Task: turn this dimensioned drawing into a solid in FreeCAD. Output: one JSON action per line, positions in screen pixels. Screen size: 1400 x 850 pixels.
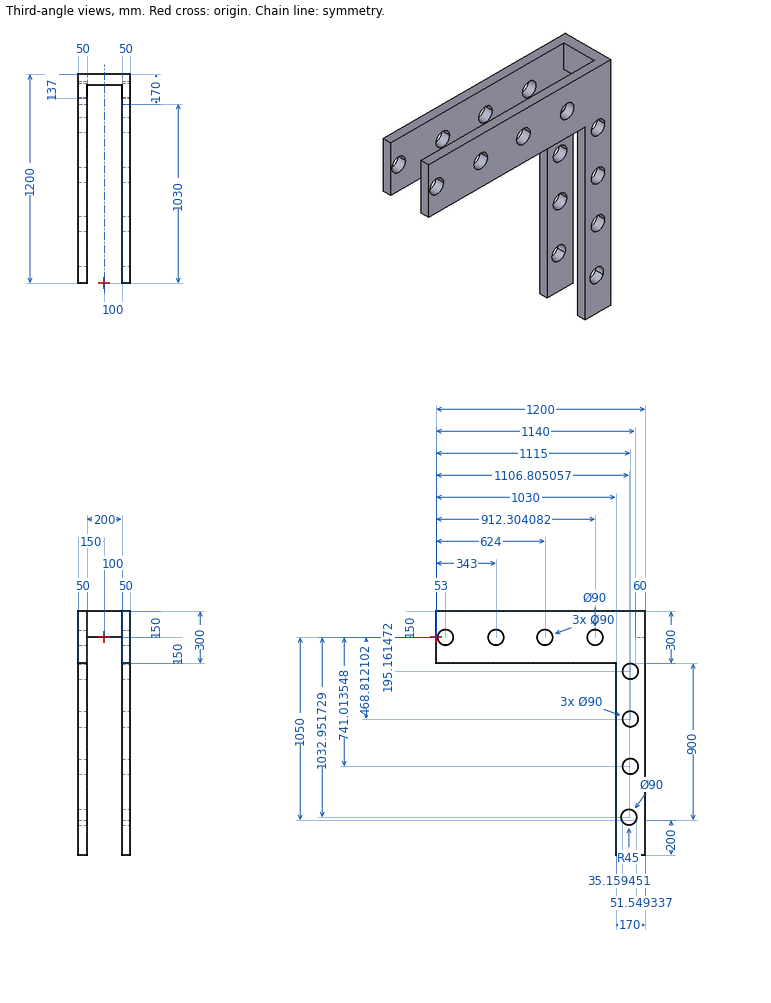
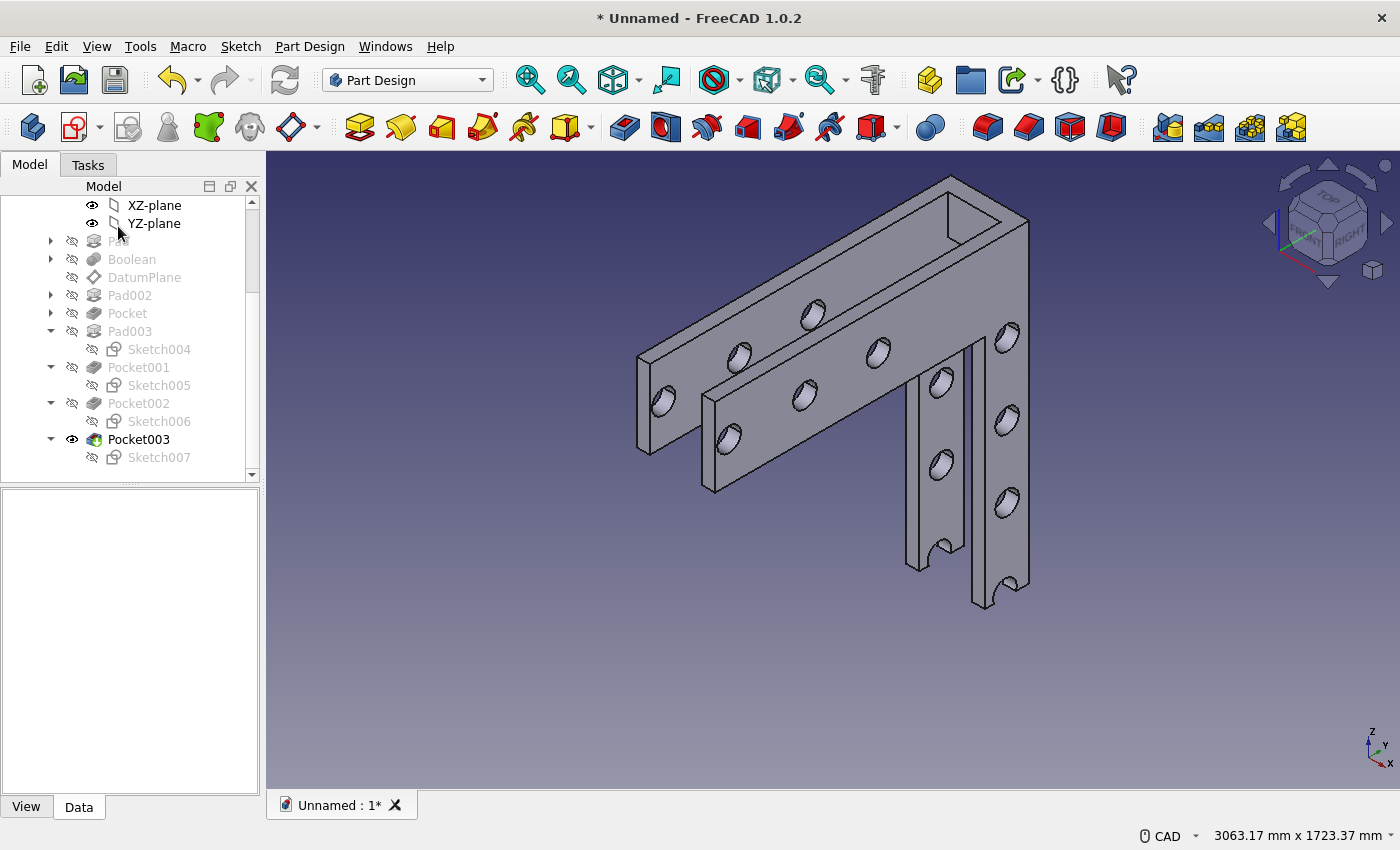
{"action": "key", "text": "6"}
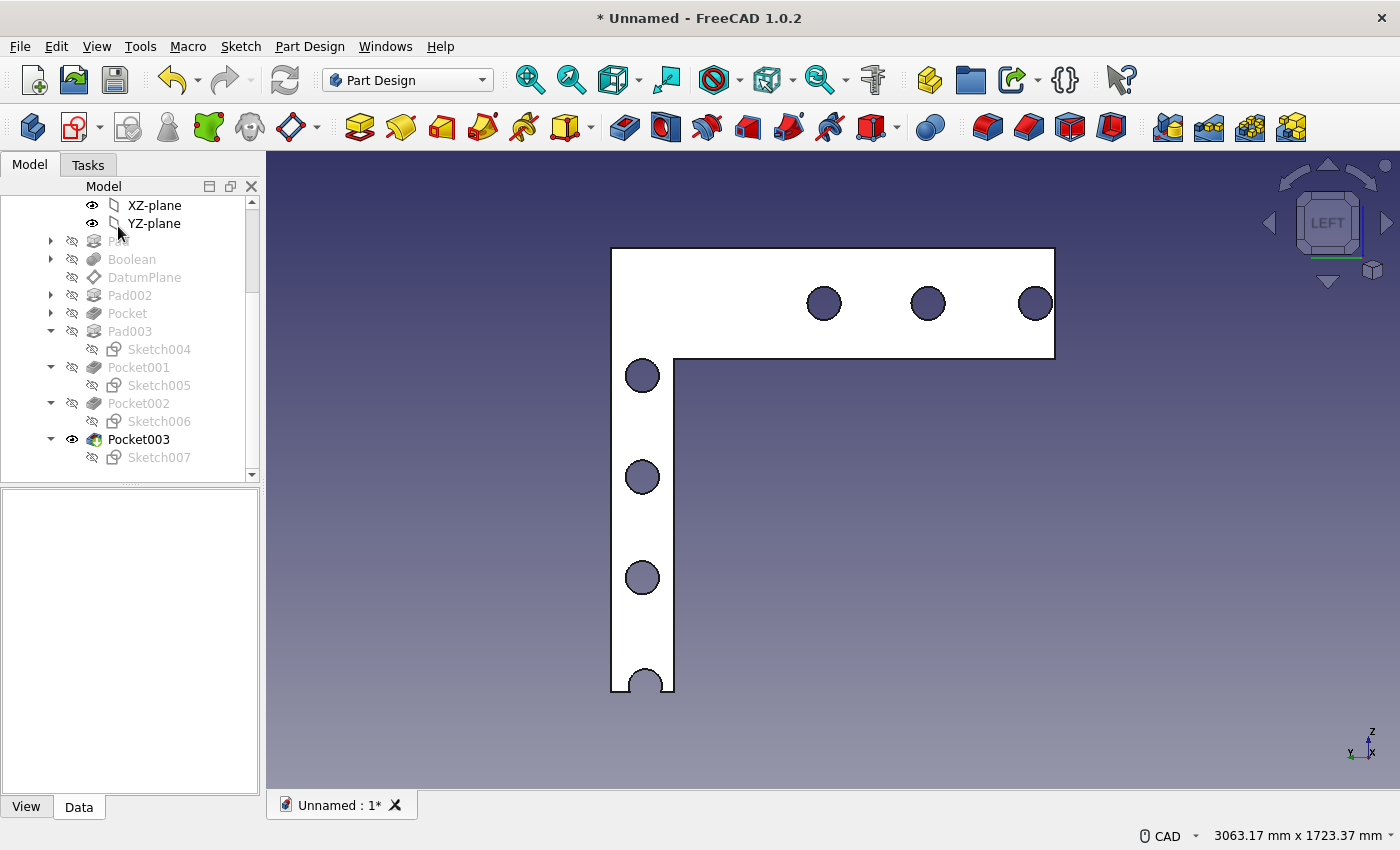
{"action": "left_click", "coordinate": [770, 279]}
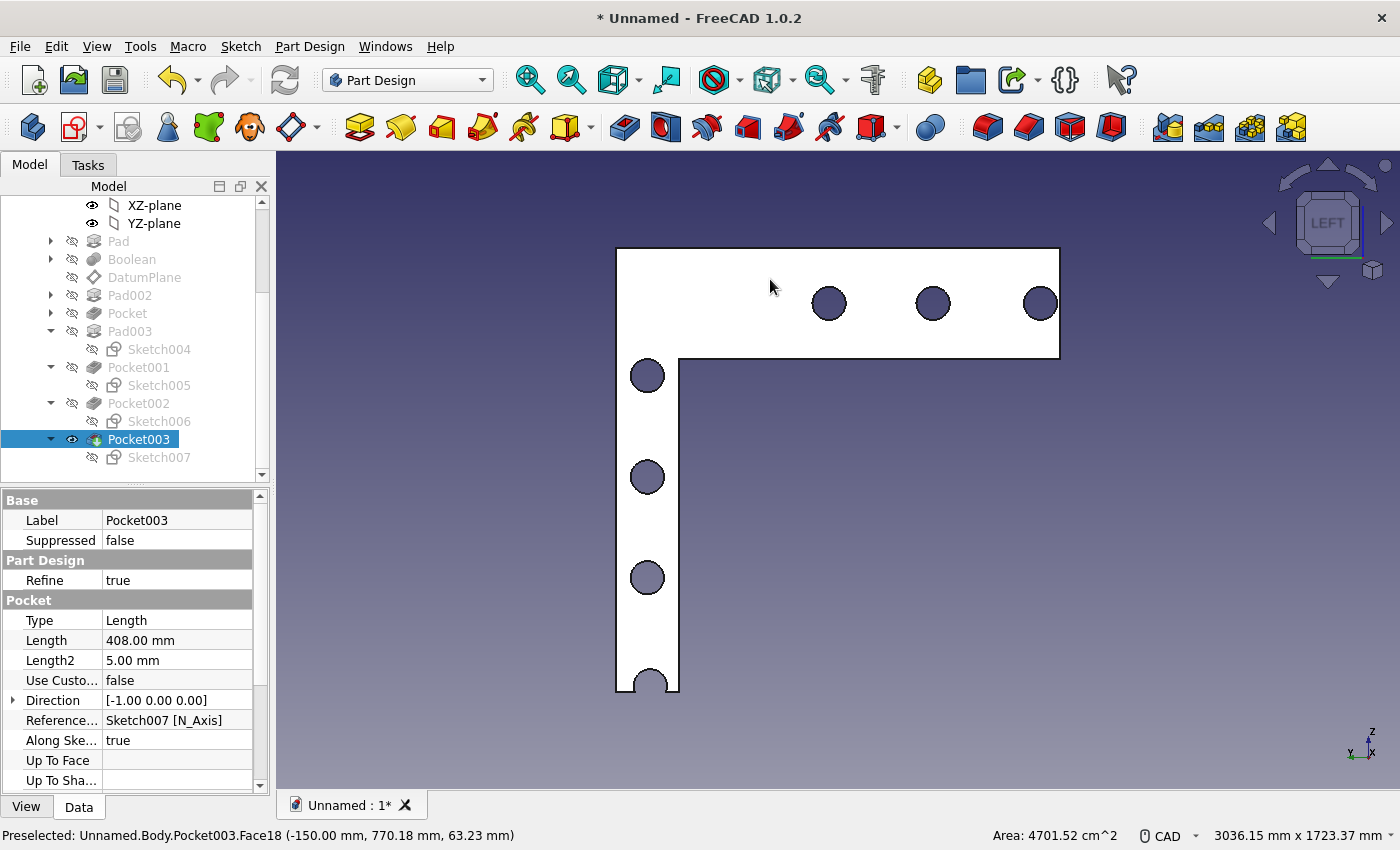
{"action": "left_click", "coordinate": [74, 128]}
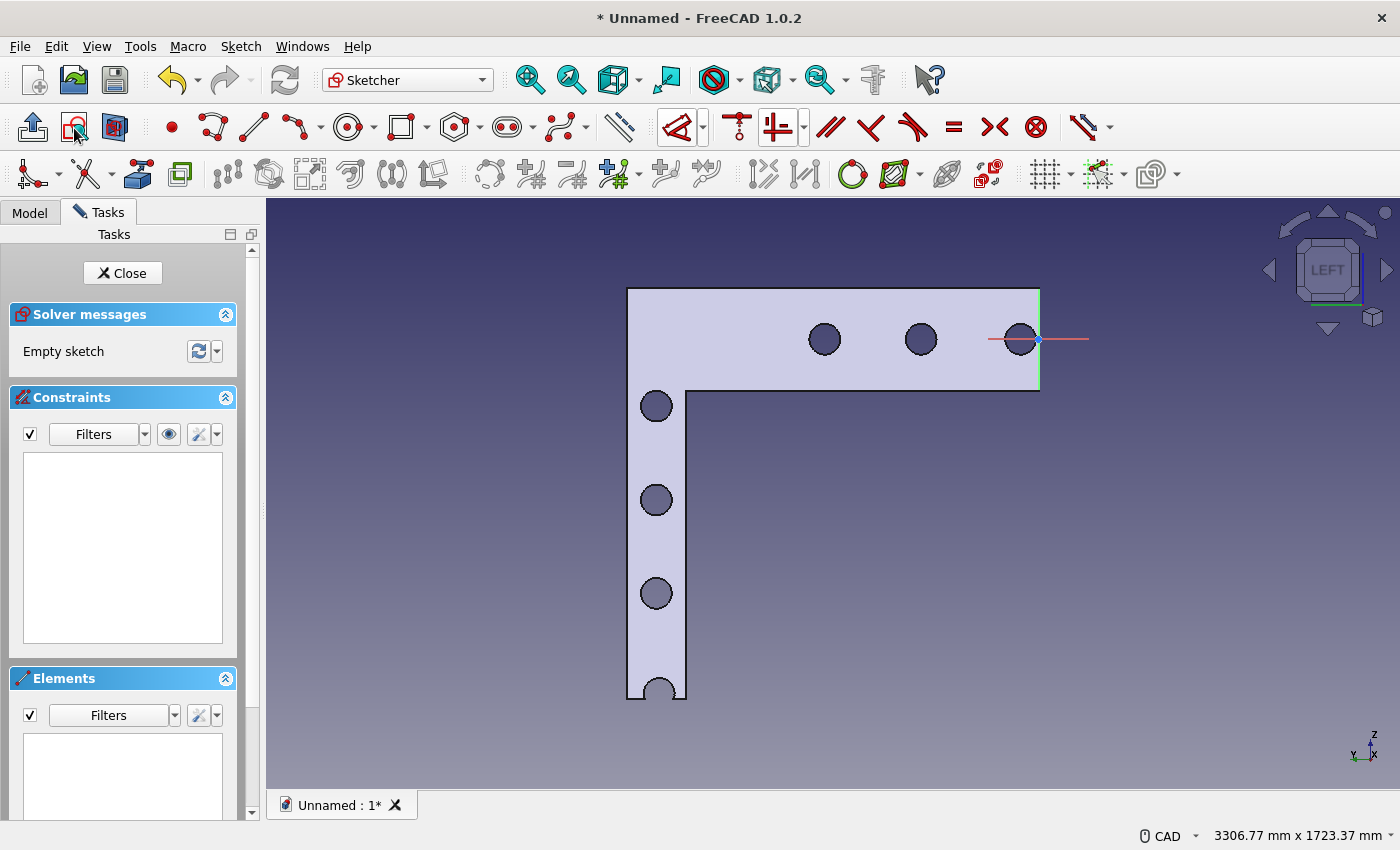
{"action": "scroll", "coordinate": [723, 327], "scroll_direction": "up", "scroll_amount": 13}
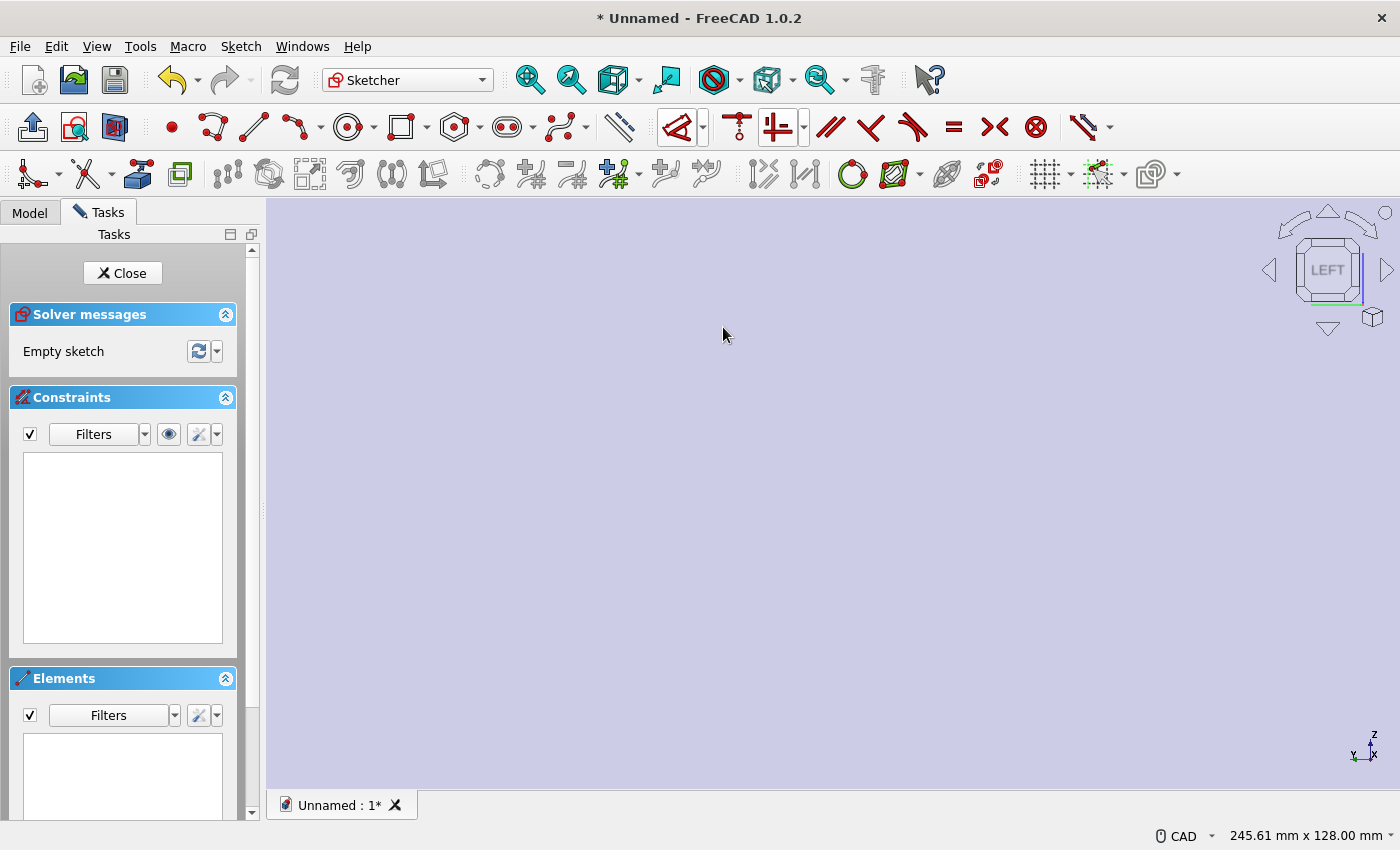
{"action": "left_click", "coordinate": [348, 128]}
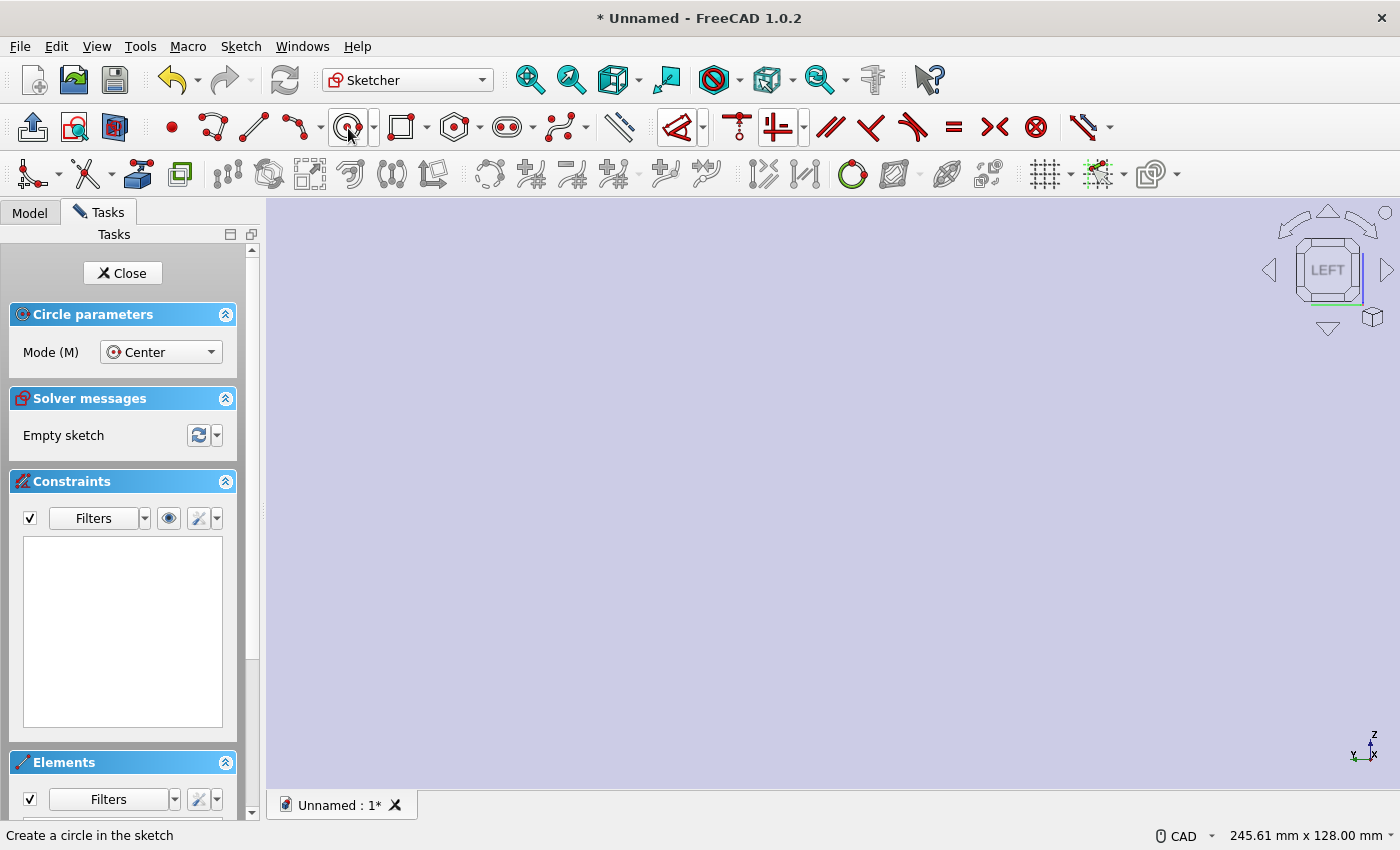
{"action": "left_click", "coordinate": [757, 488]}
{"action": "left_click", "coordinate": [904, 341]}
{"action": "key", "text": "Escape"}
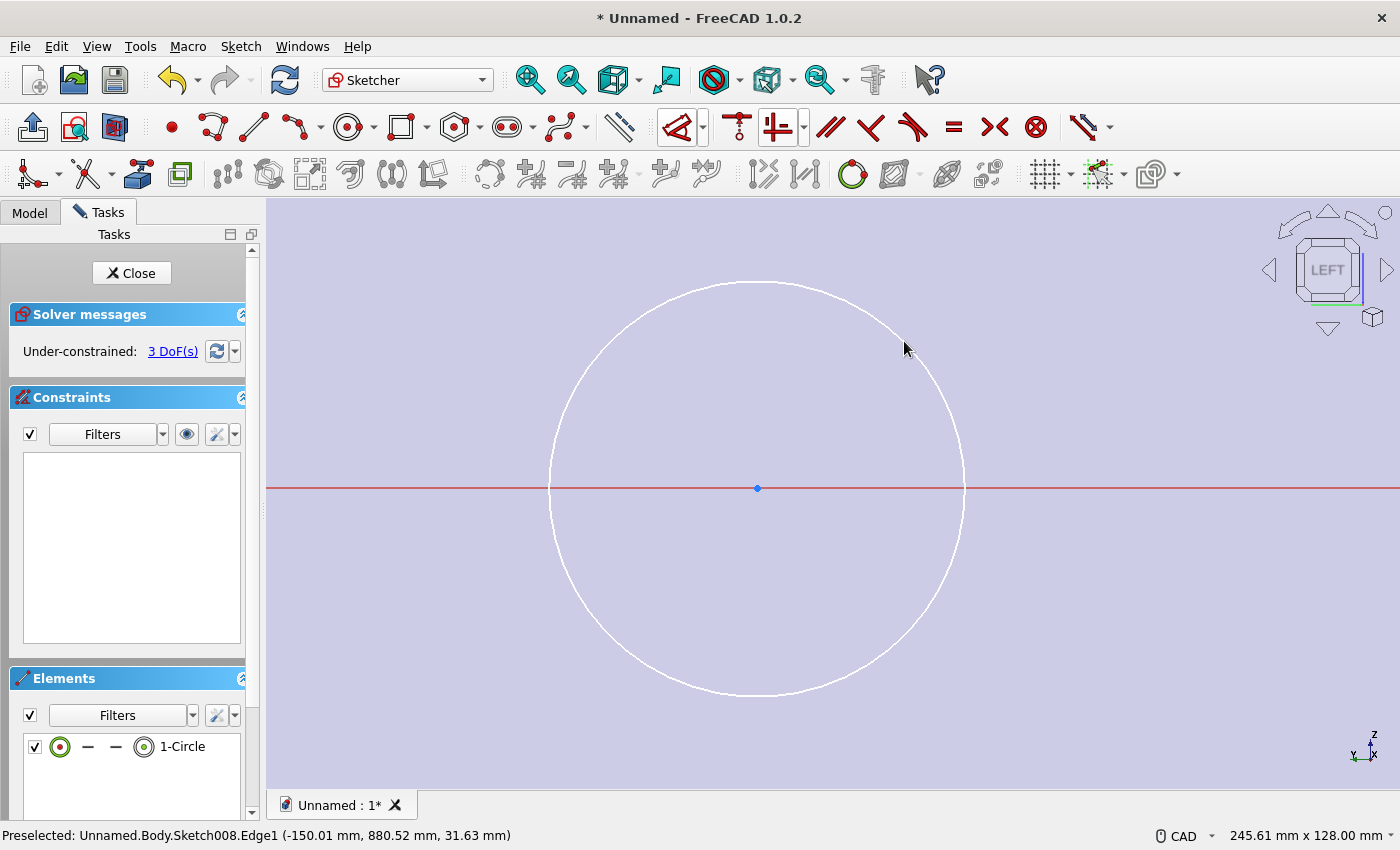
{"action": "left_click", "coordinate": [757, 489]}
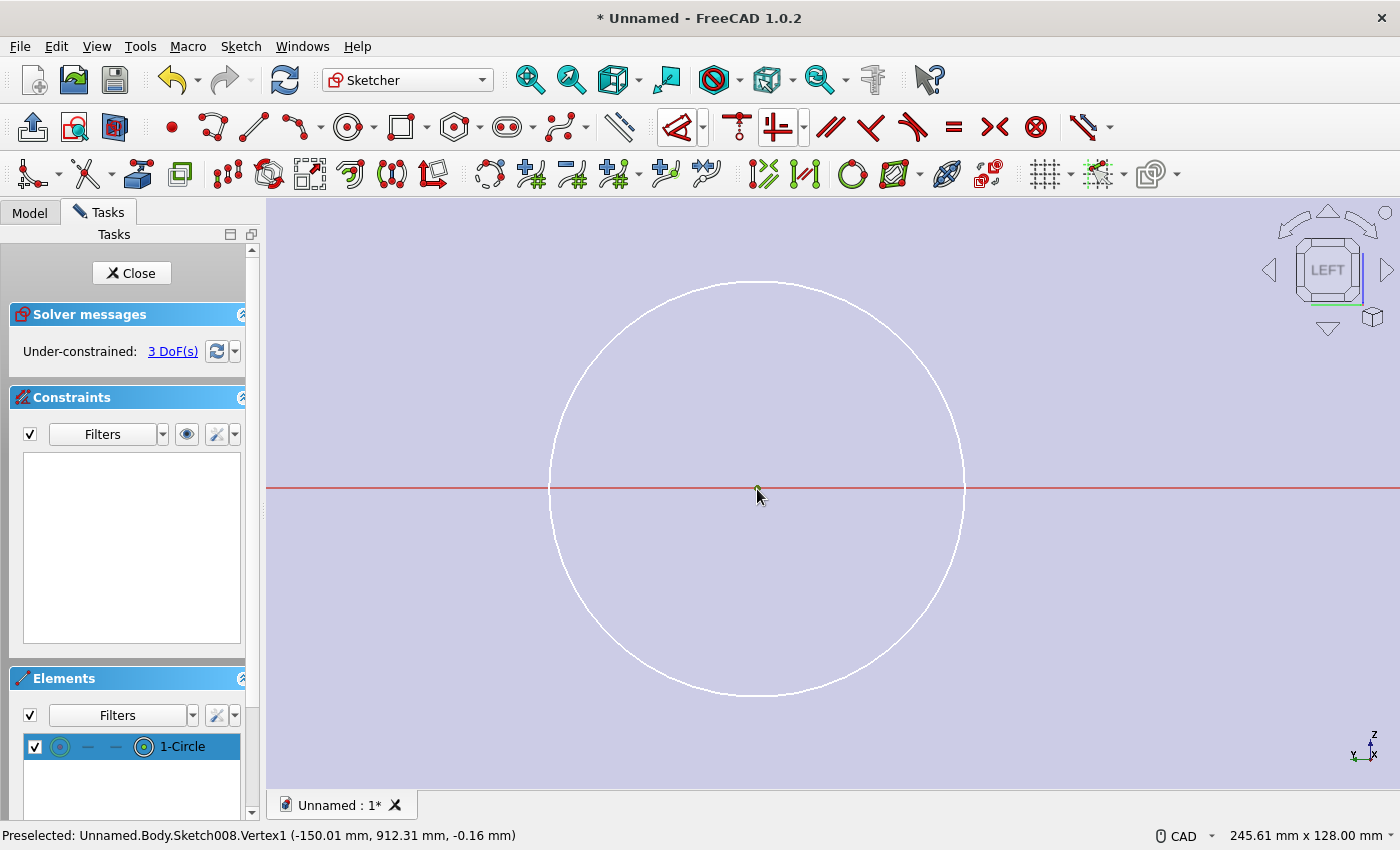
{"action": "left_click", "coordinate": [361, 488]}